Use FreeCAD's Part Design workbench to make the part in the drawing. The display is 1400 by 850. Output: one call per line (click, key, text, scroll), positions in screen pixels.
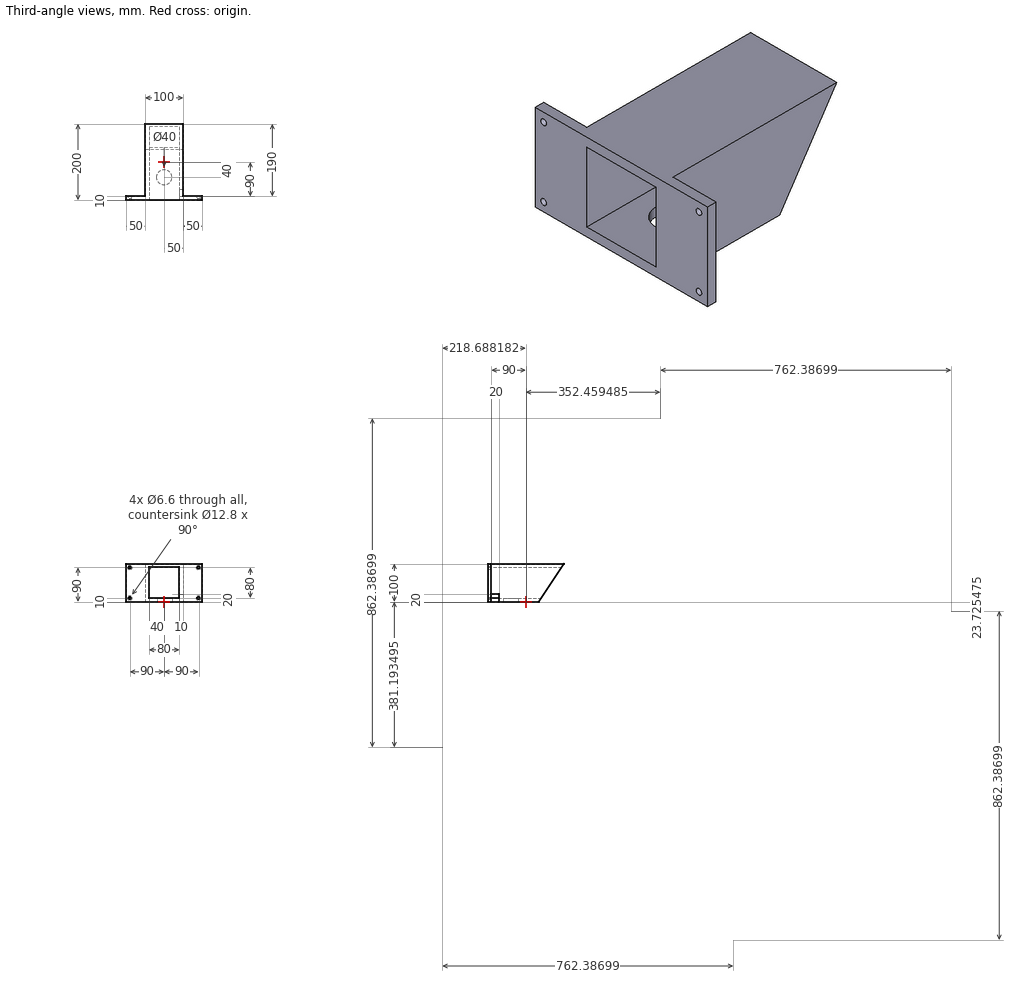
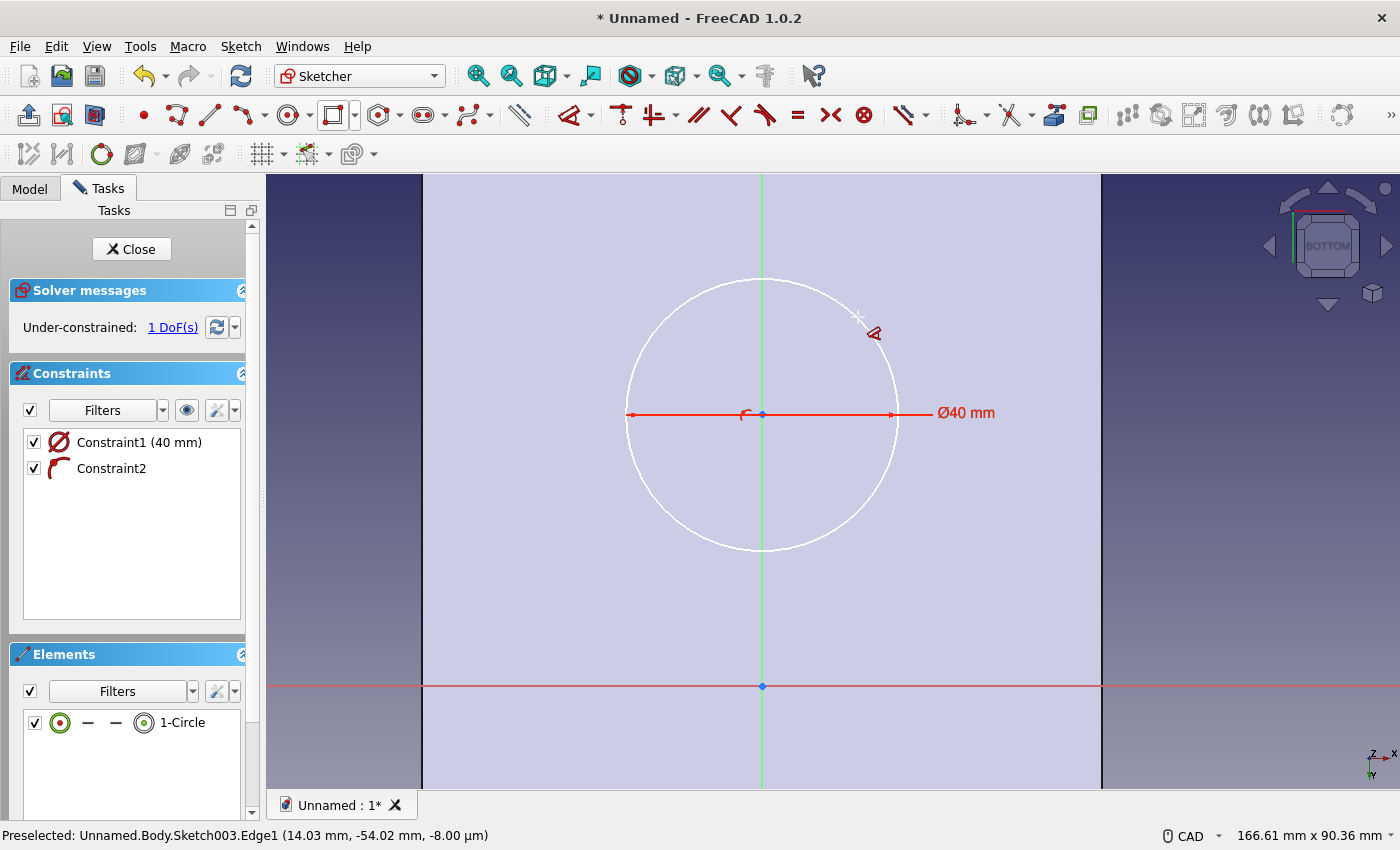
click(762, 415)
click(796, 488)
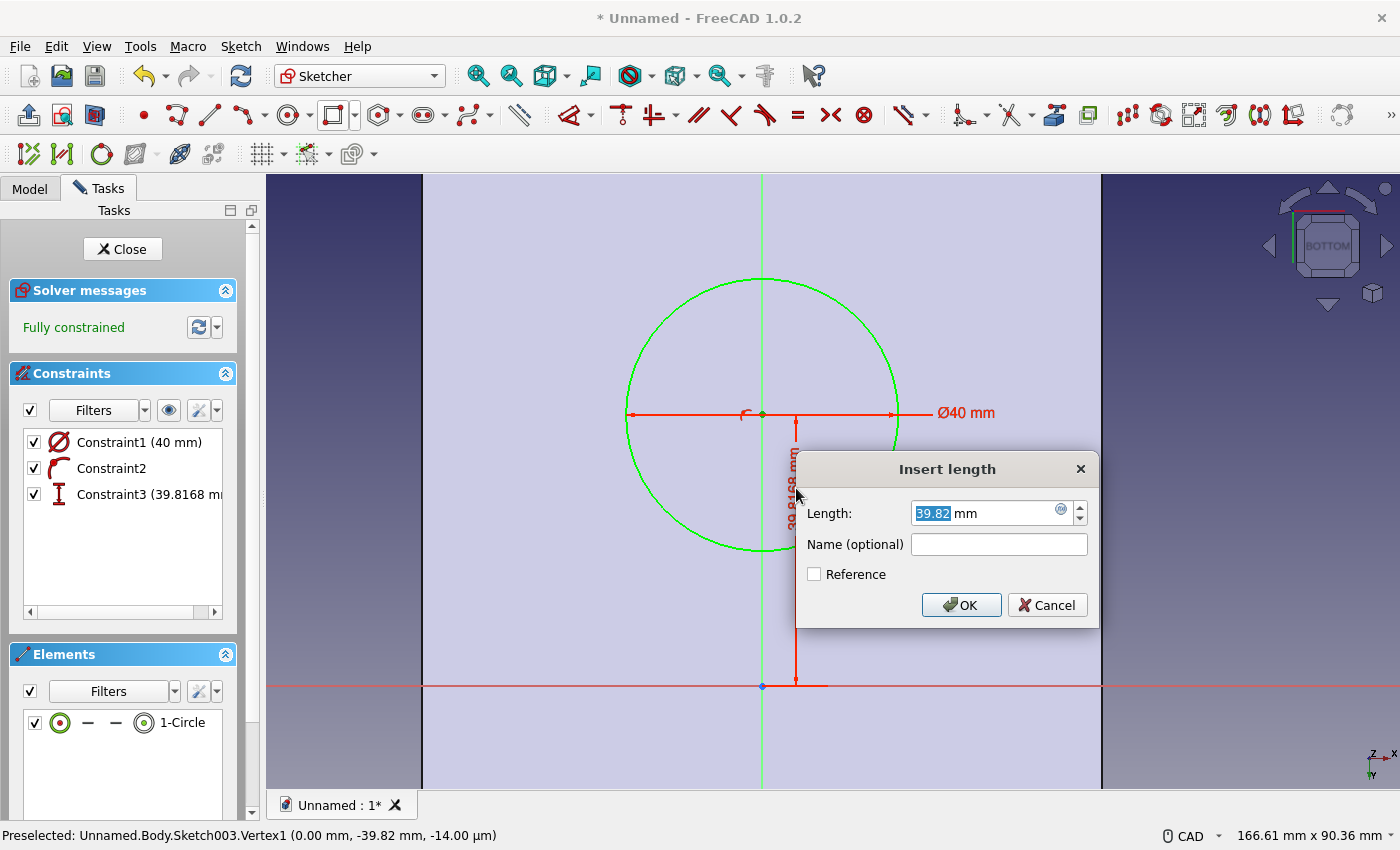
text(40)
key(Return)
key(Escape)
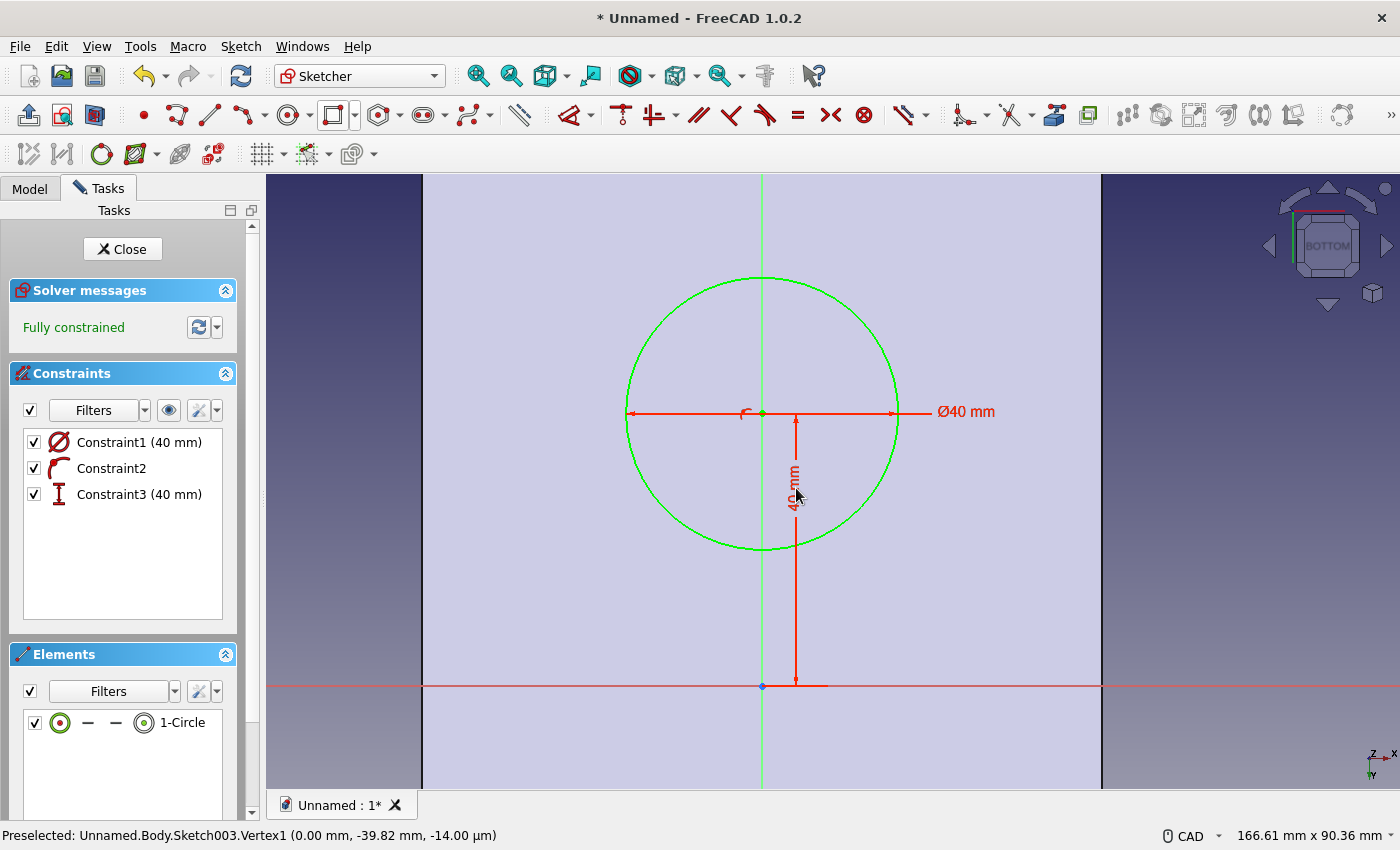
click(123, 249)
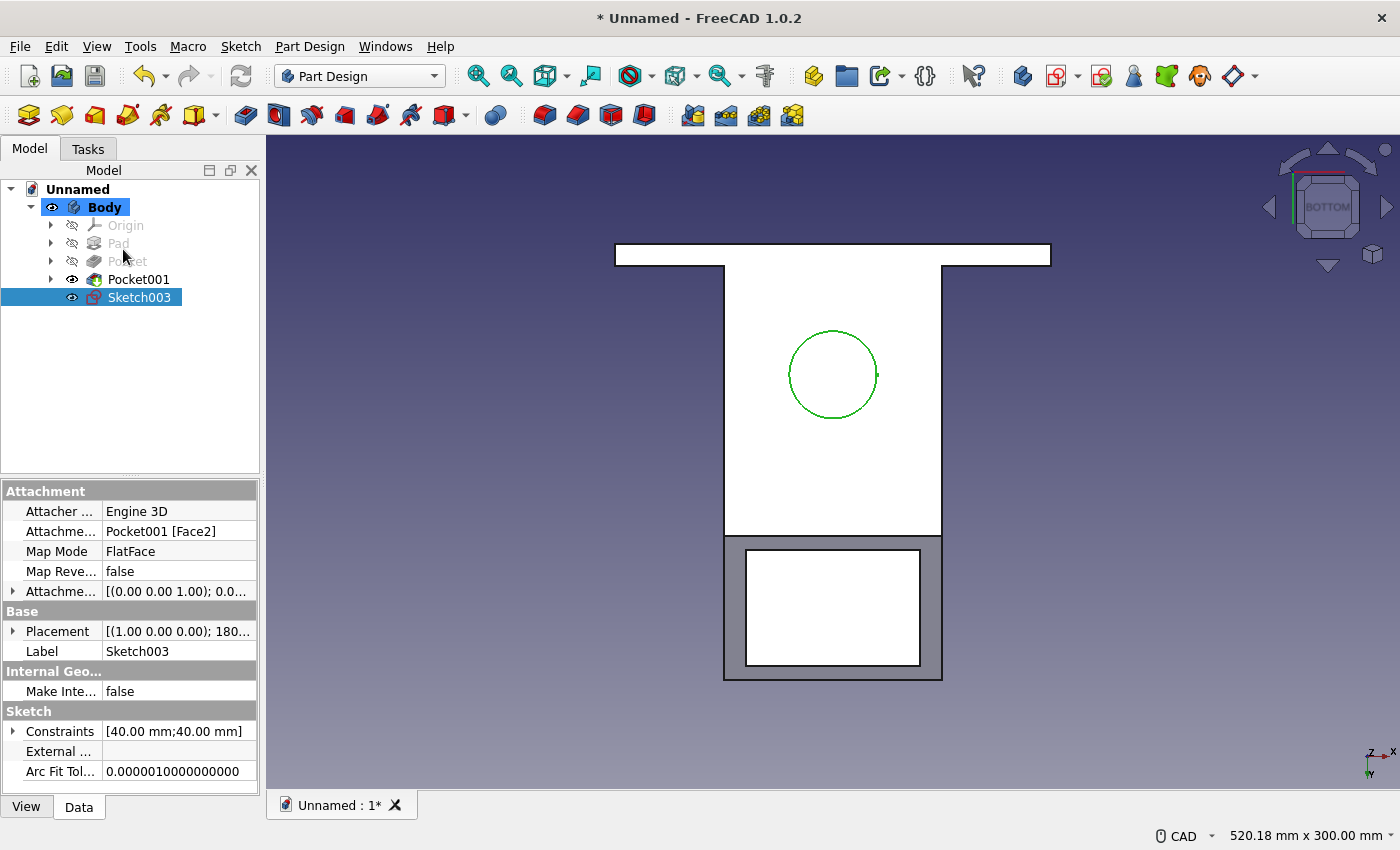
click(246, 116)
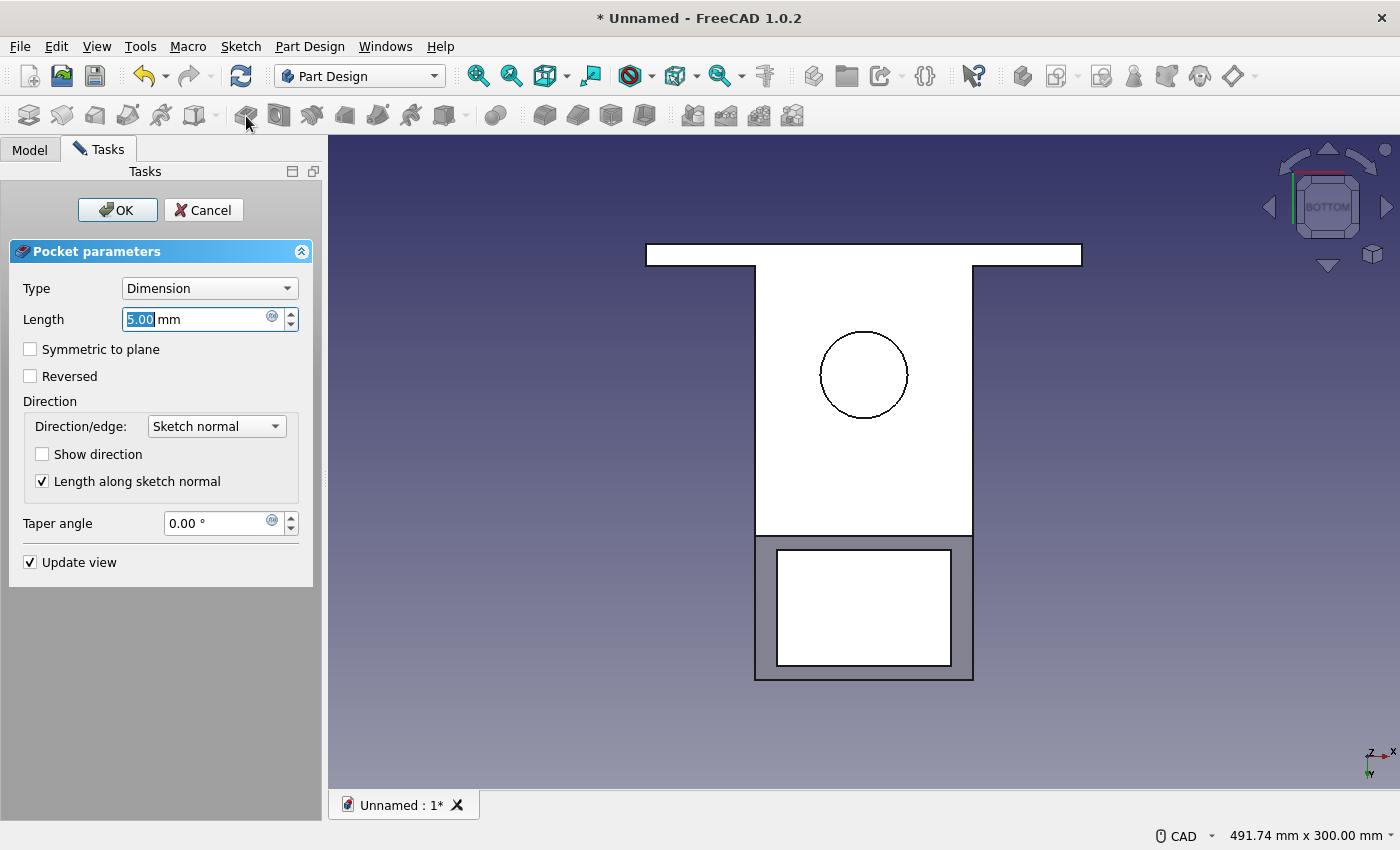
text(20)
key(Tab)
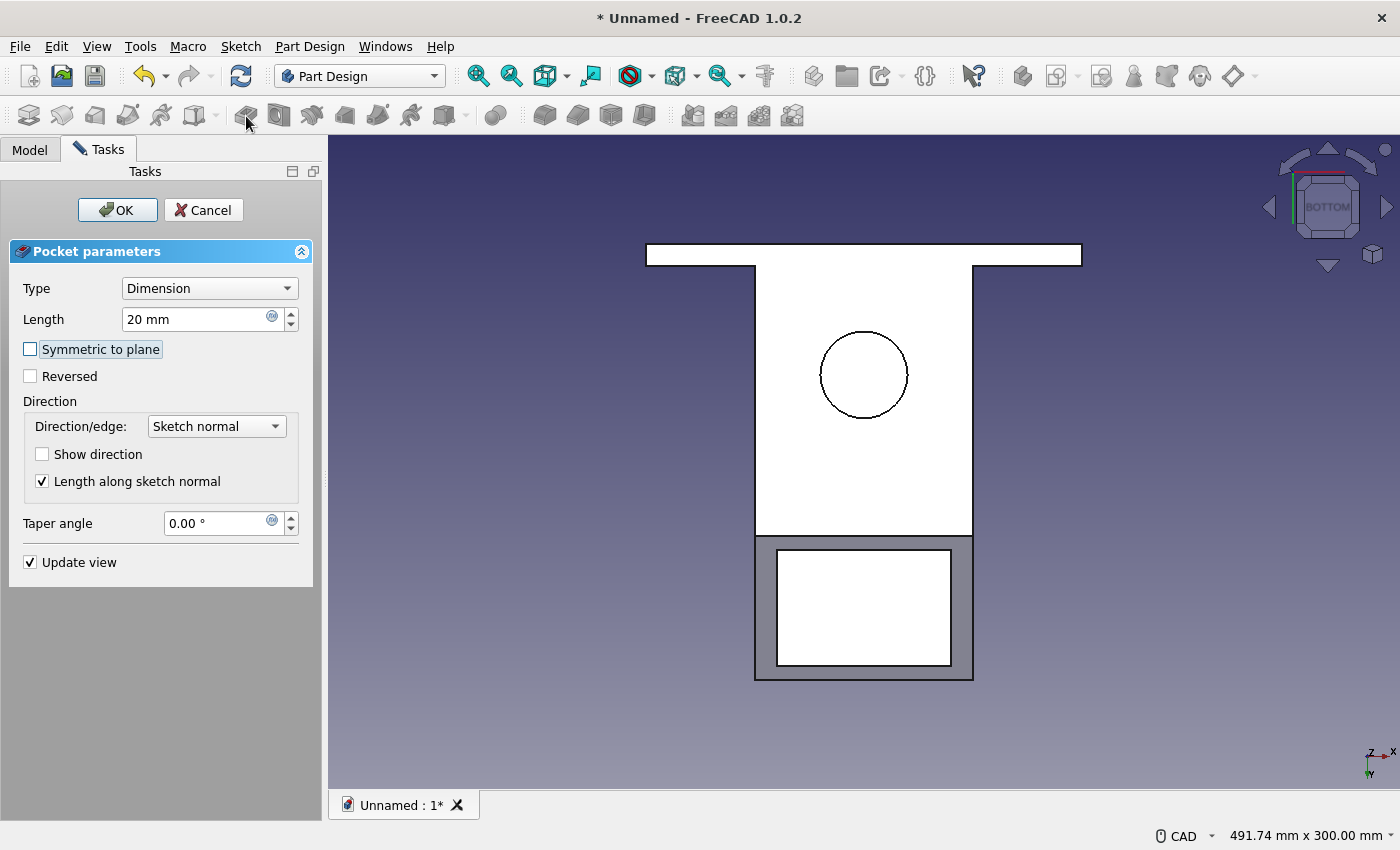
click(118, 210)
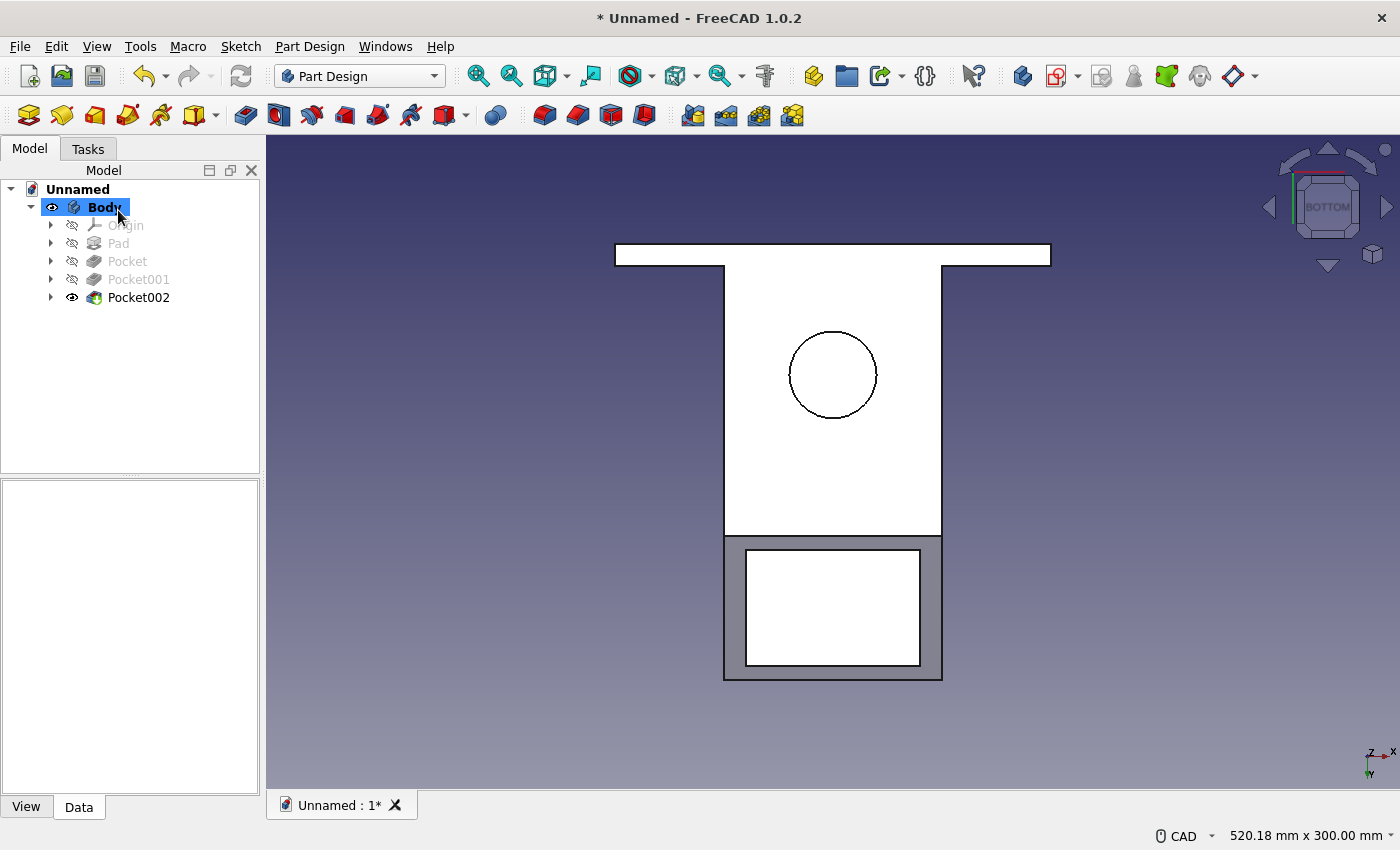
key(4)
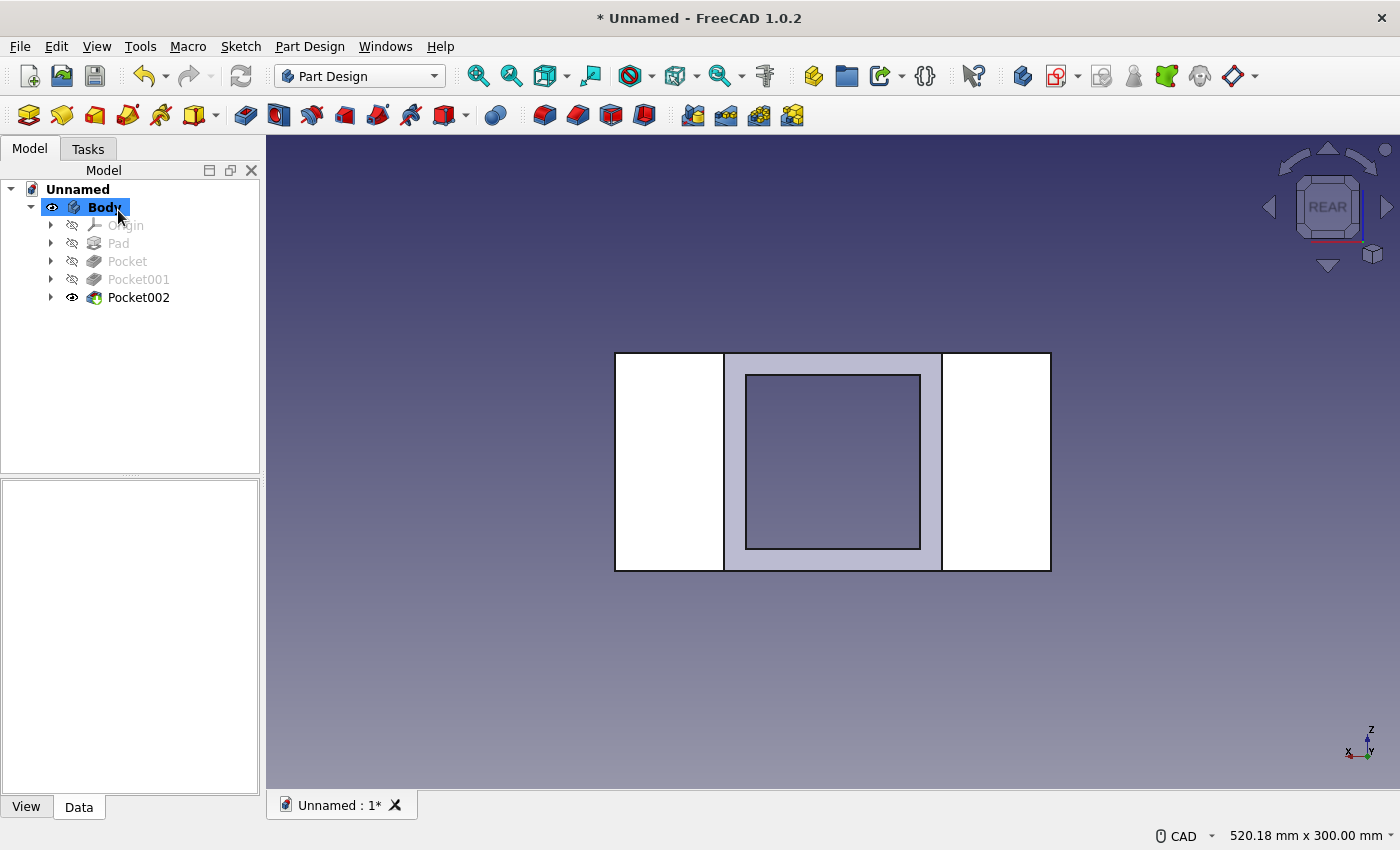
key(v)
key(f)